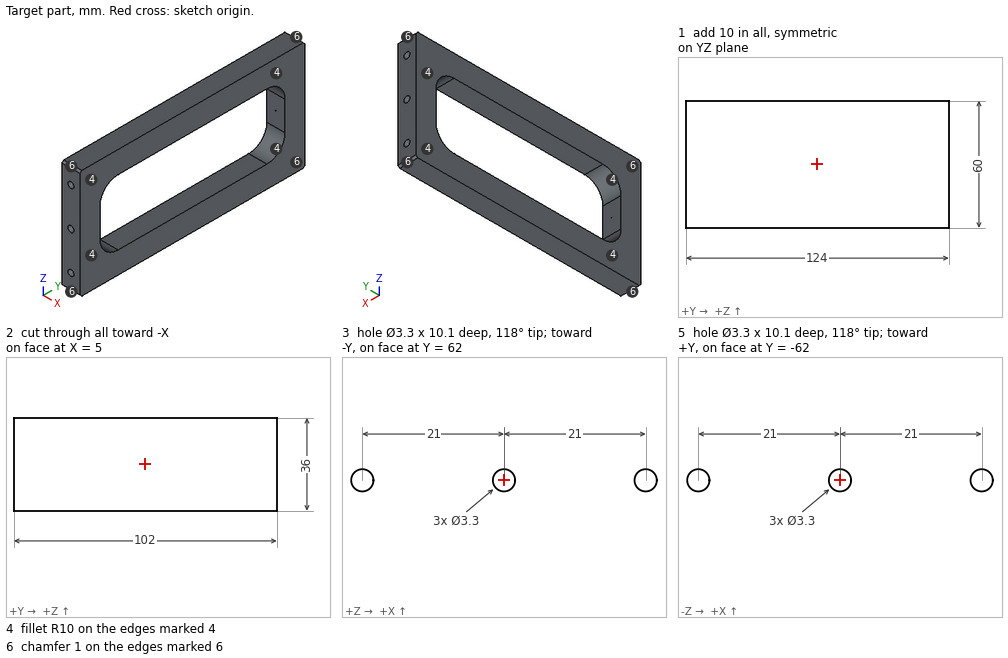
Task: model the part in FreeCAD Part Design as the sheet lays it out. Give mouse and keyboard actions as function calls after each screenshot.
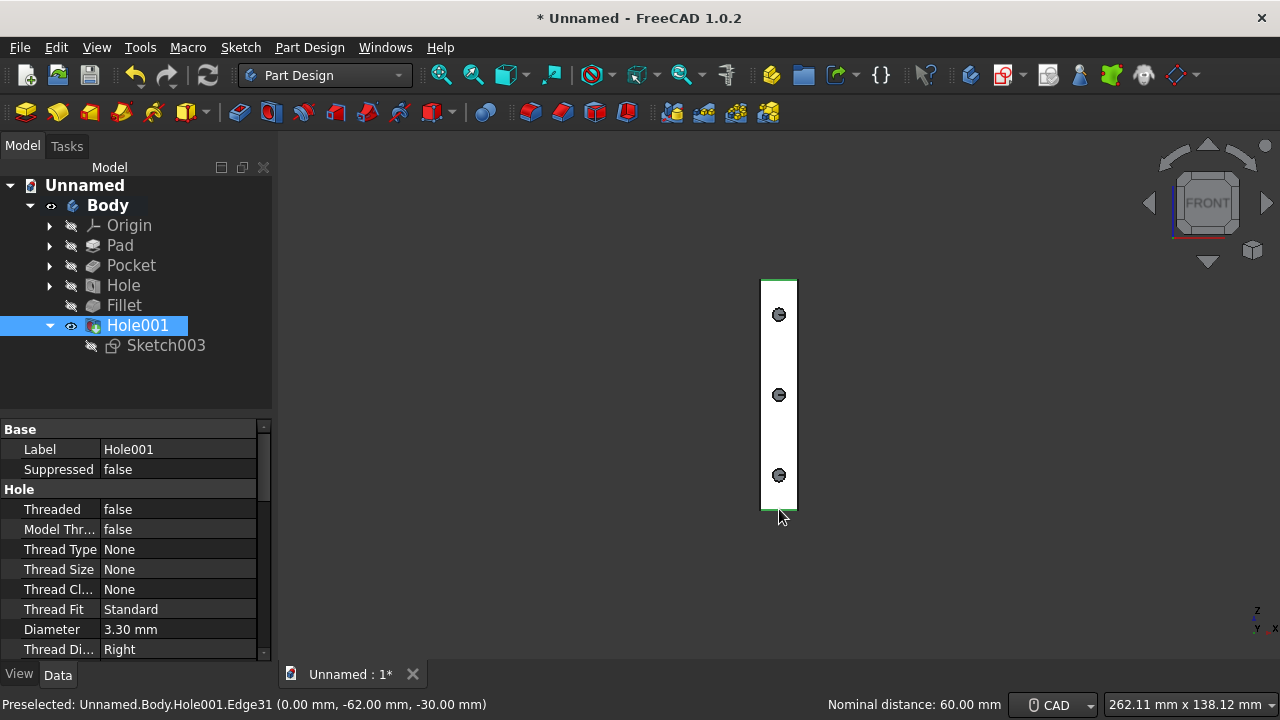
key(3)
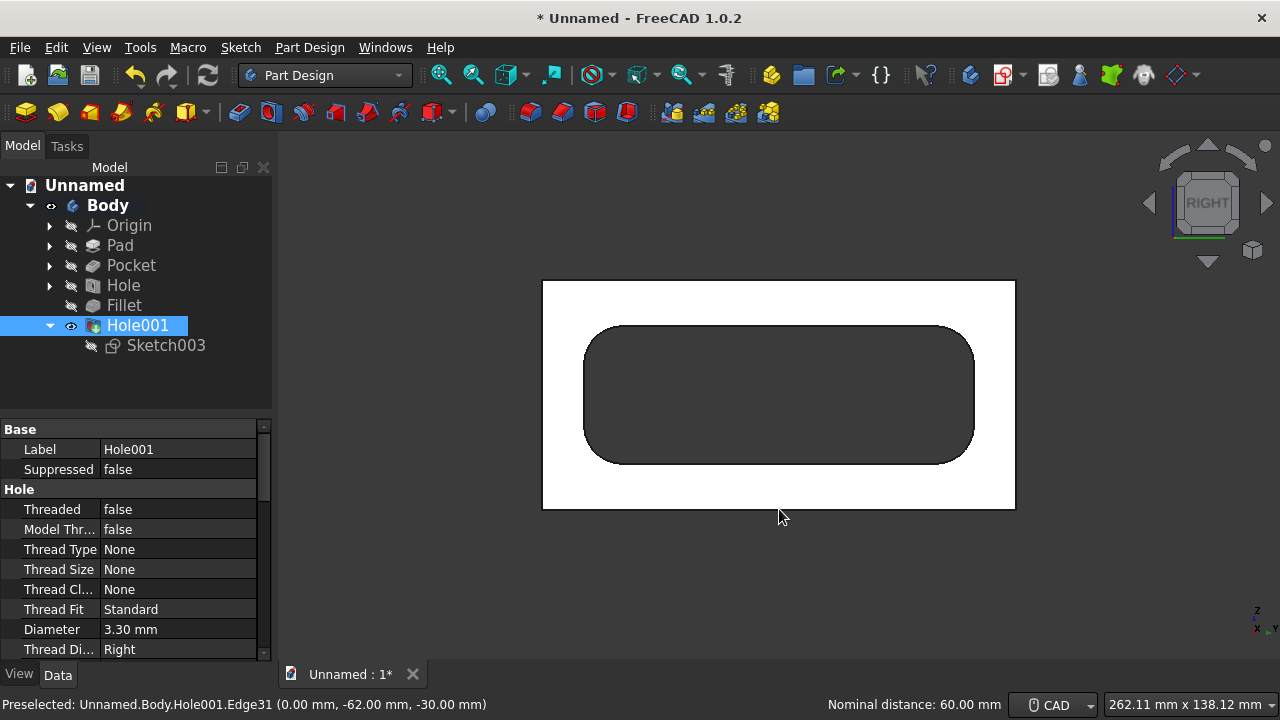
key(5)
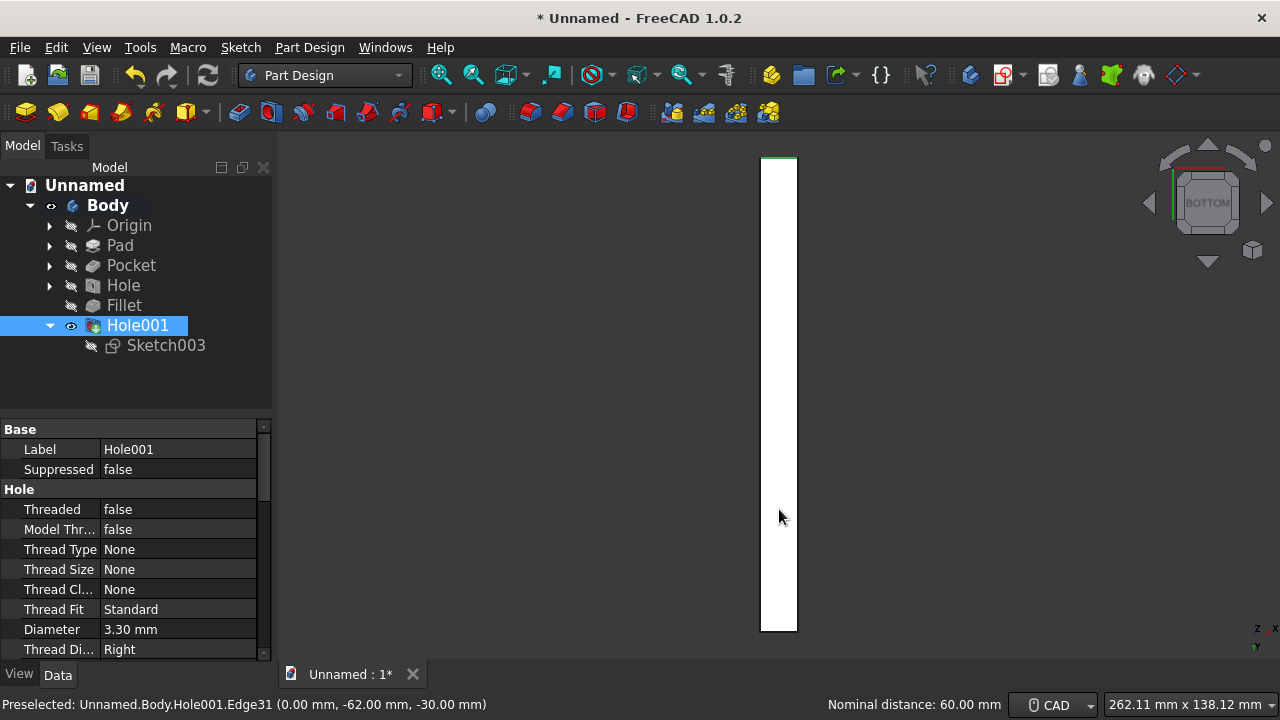
key(4)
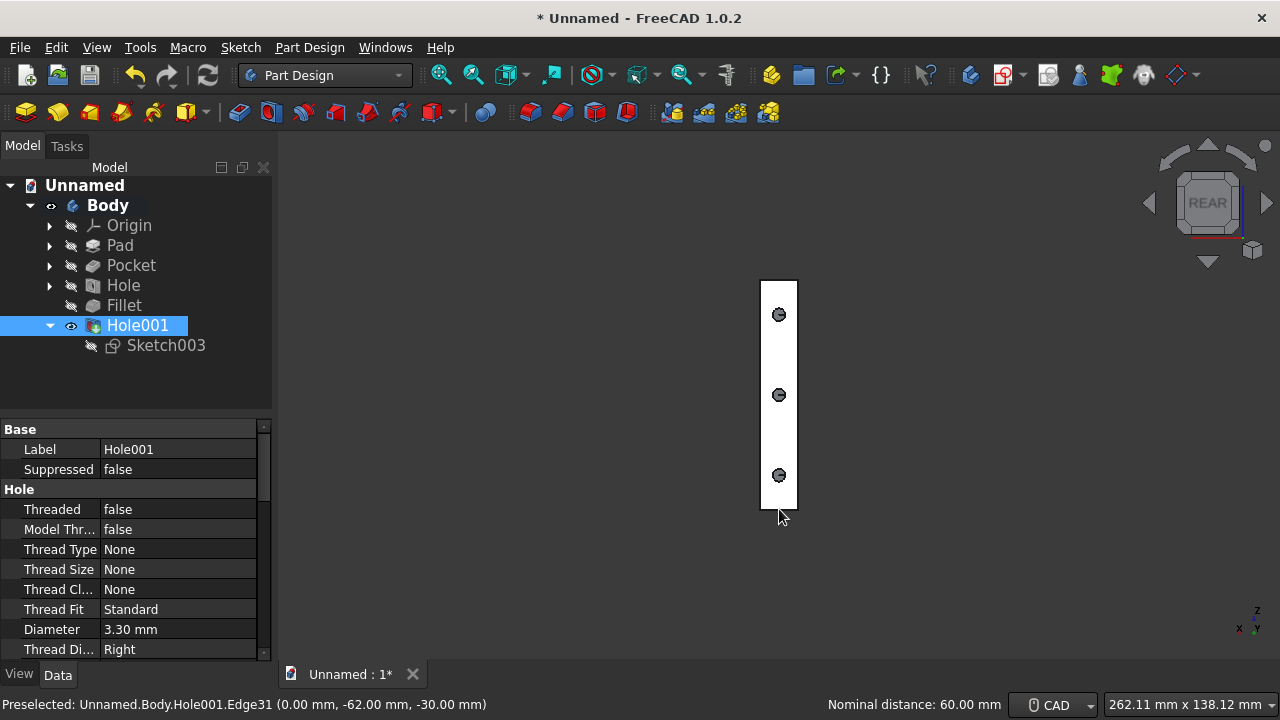
click(442, 76)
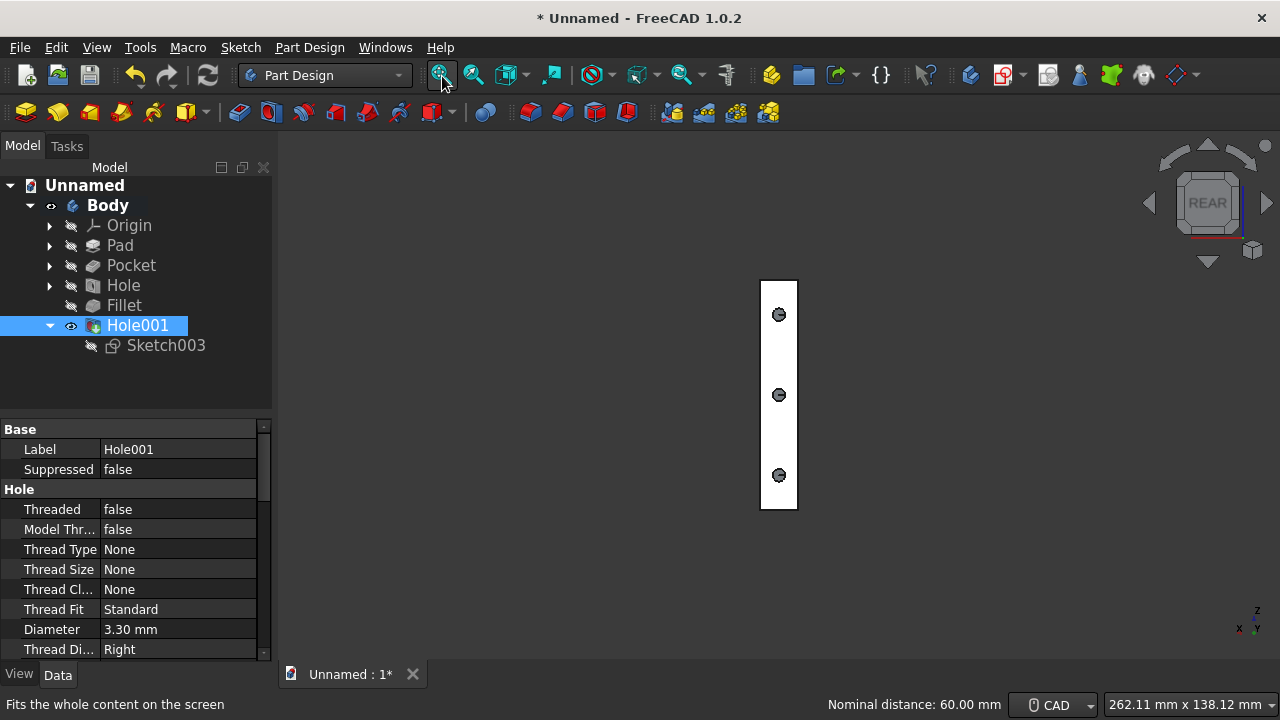
click(779, 279, ctrl)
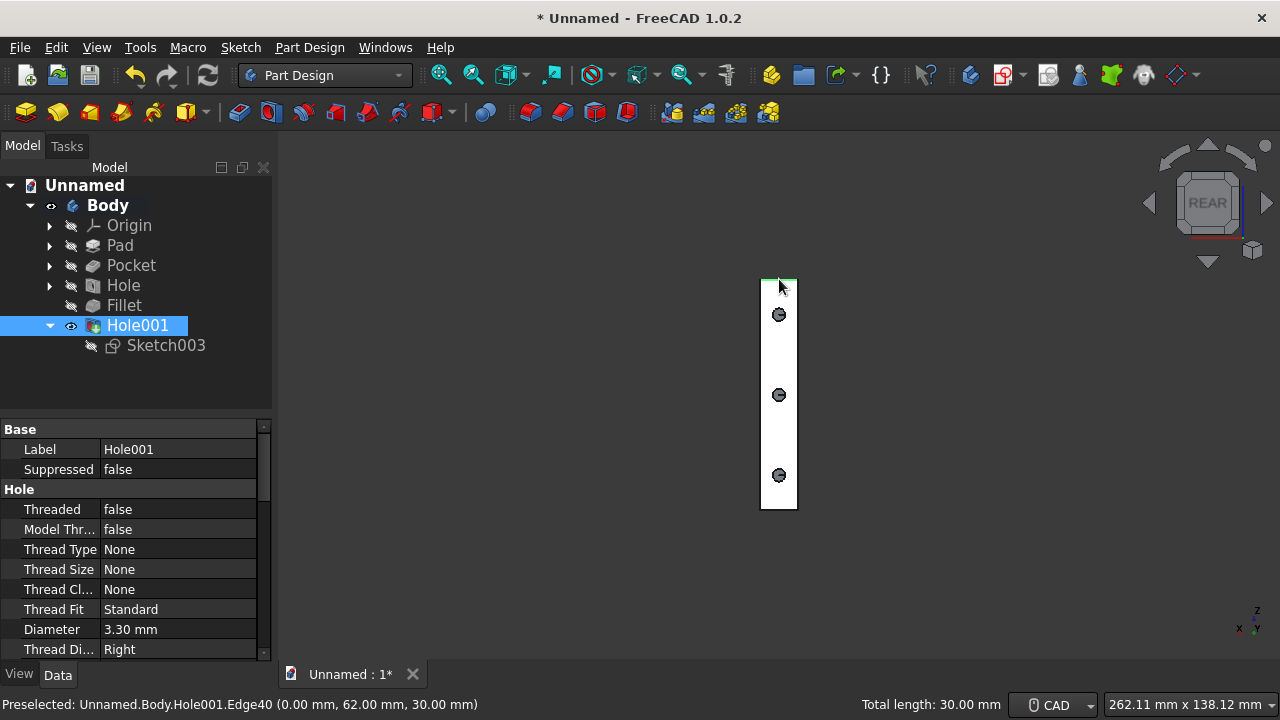
click(779, 509, ctrl)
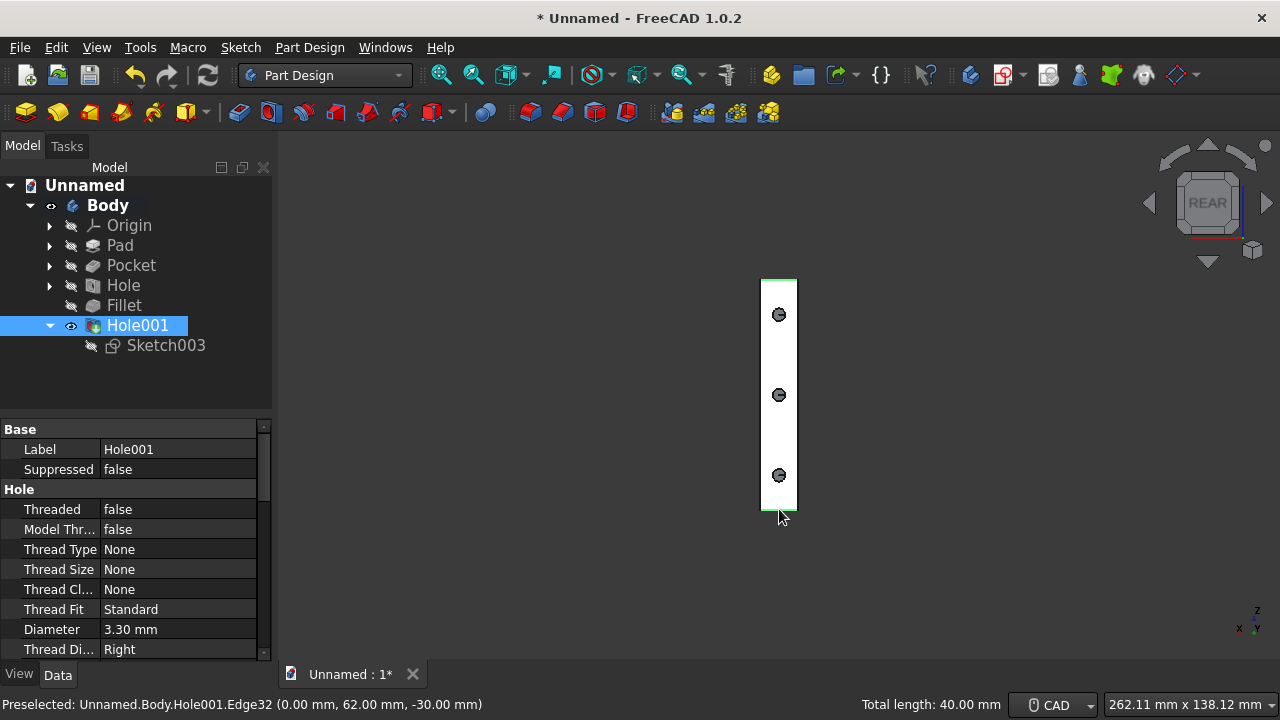
click(564, 112)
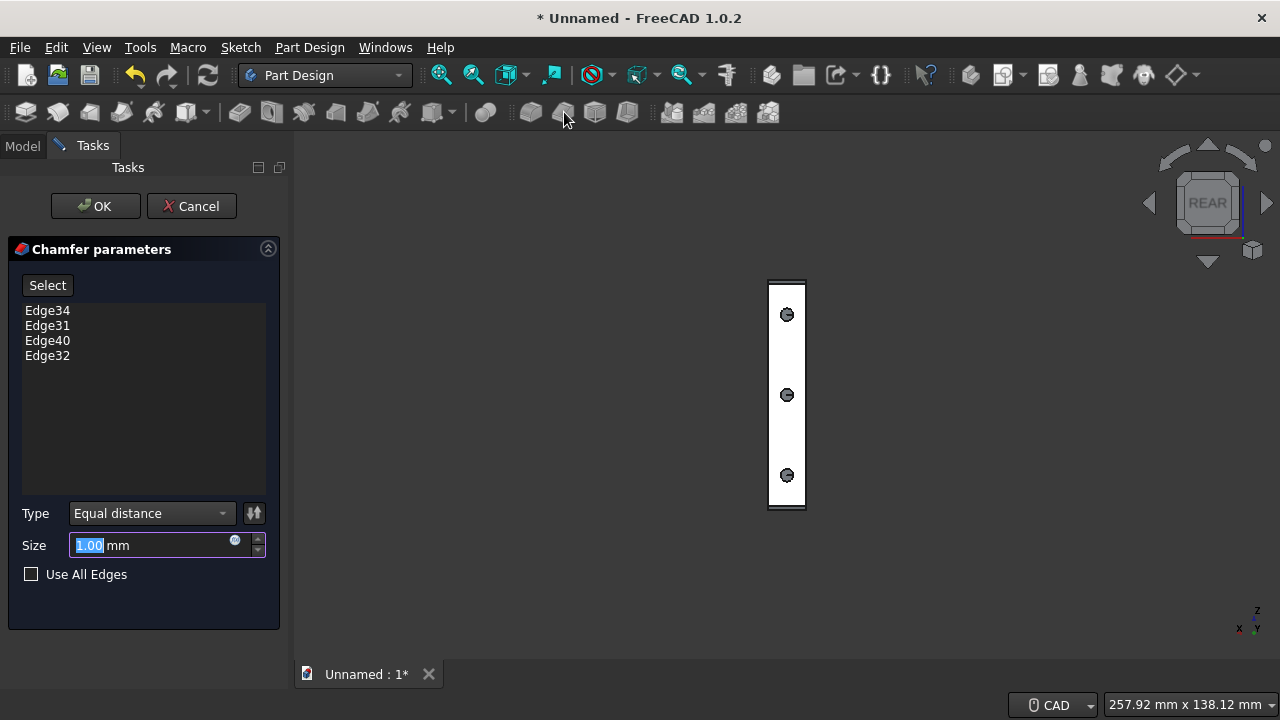
text(1)
key(Tab)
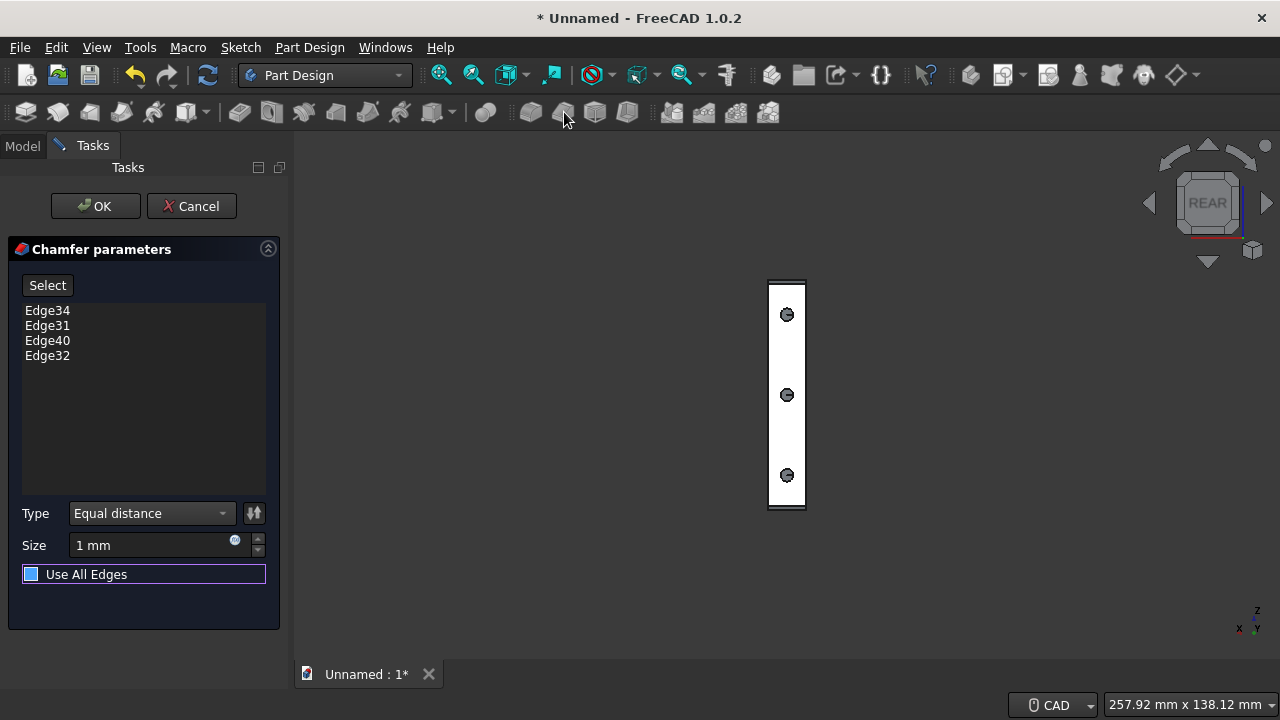
click(96, 206)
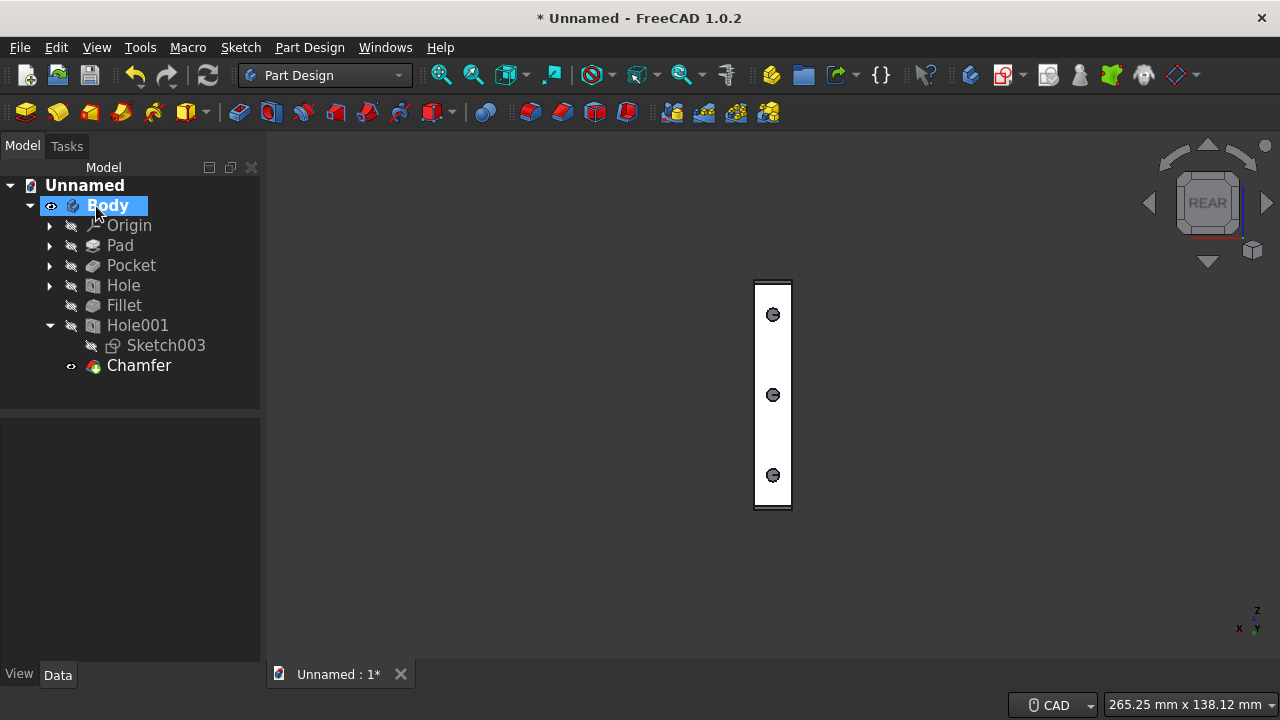
key(0)